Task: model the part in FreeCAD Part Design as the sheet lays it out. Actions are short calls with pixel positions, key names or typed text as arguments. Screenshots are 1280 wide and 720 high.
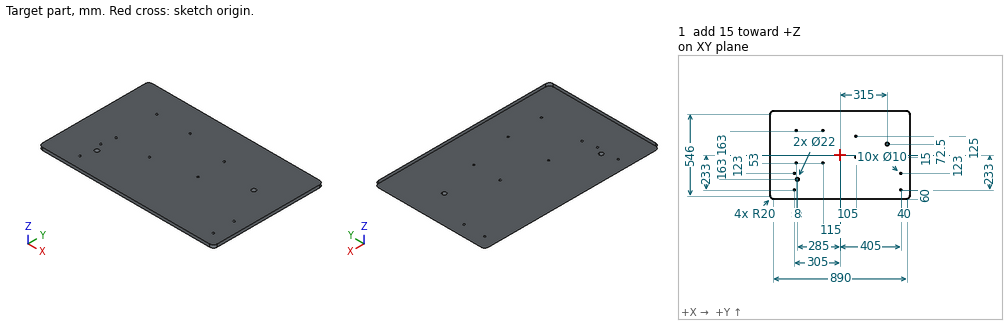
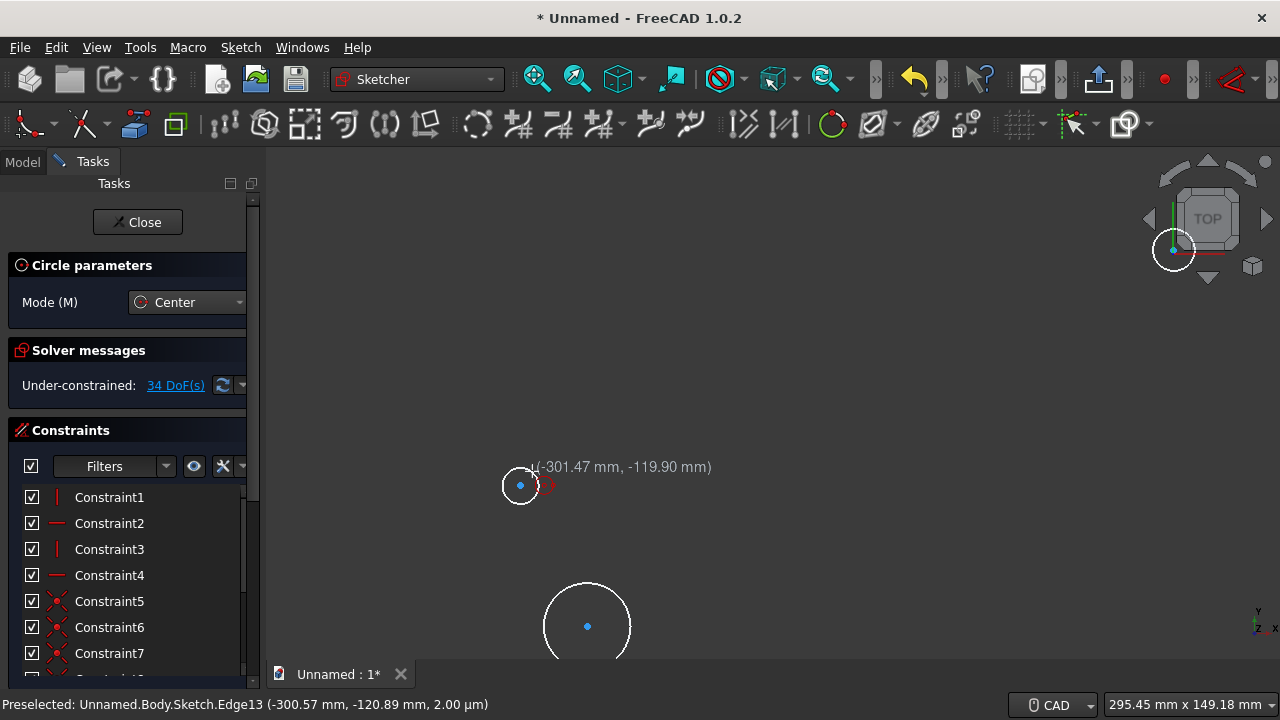
scroll(561, 242, up, 2)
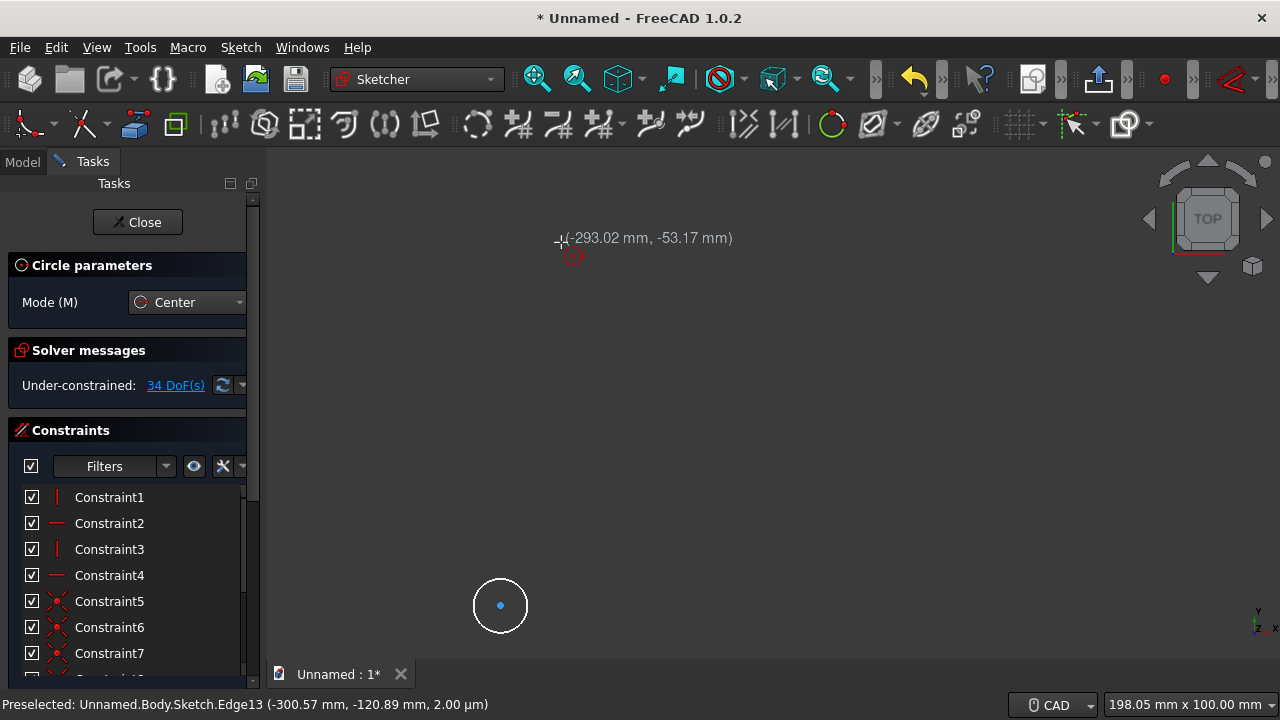
scroll(535, 457, down, 11)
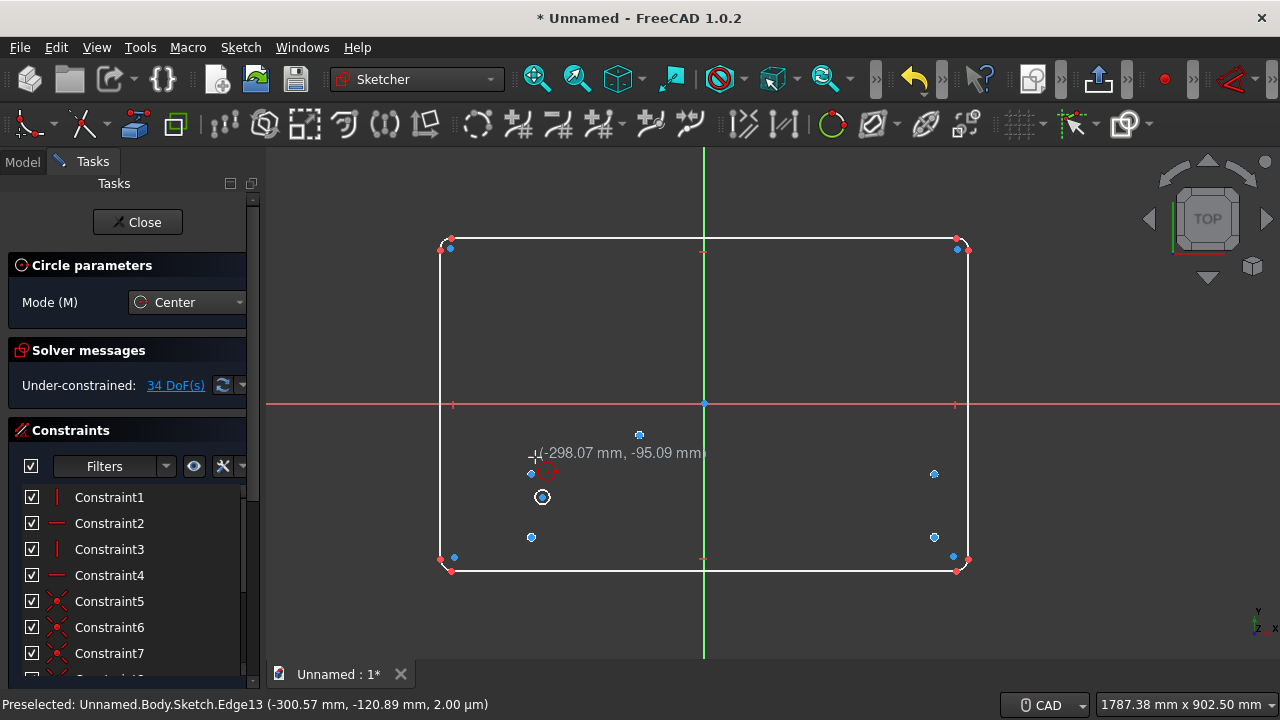
click(538, 434)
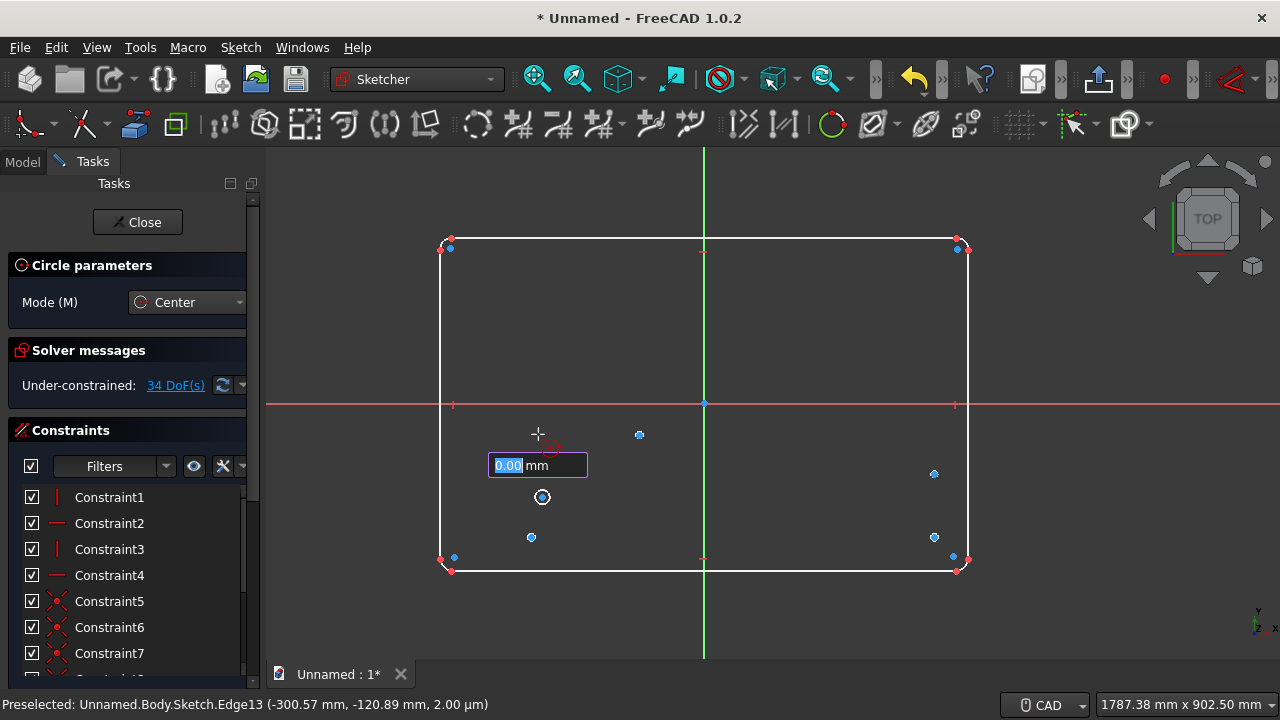
scroll(540, 432, up, 9)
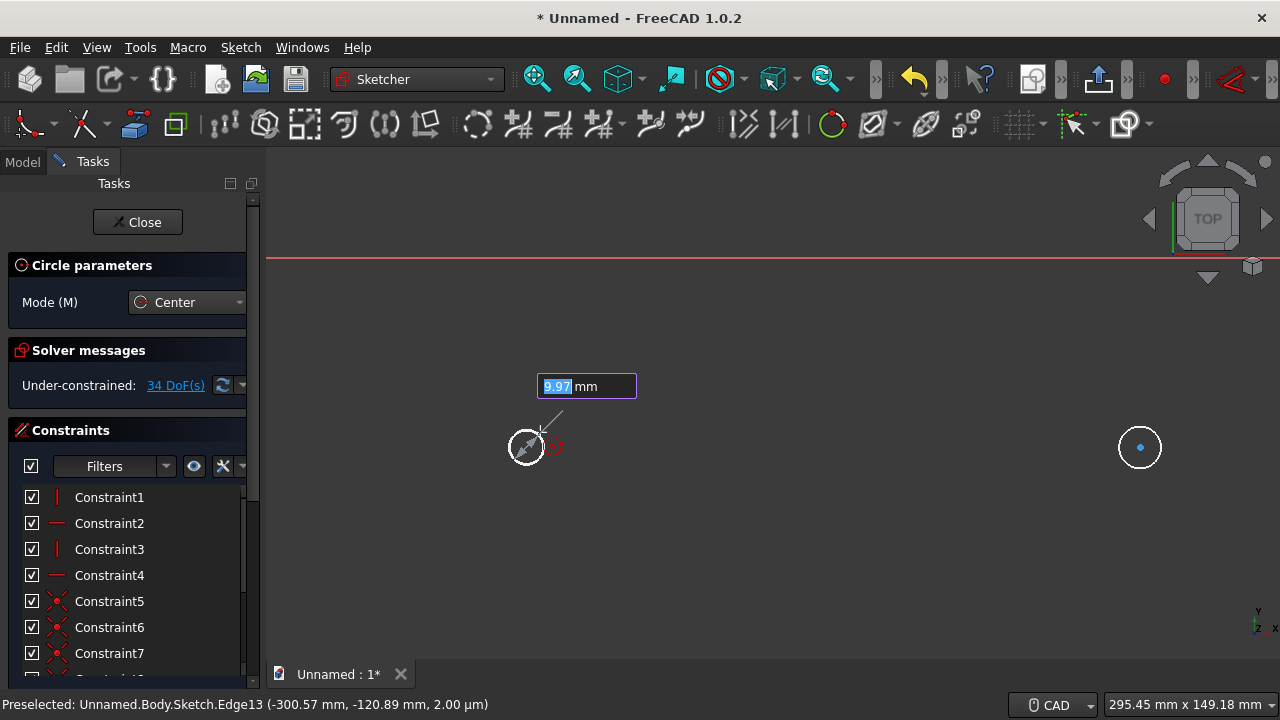
click(539, 428)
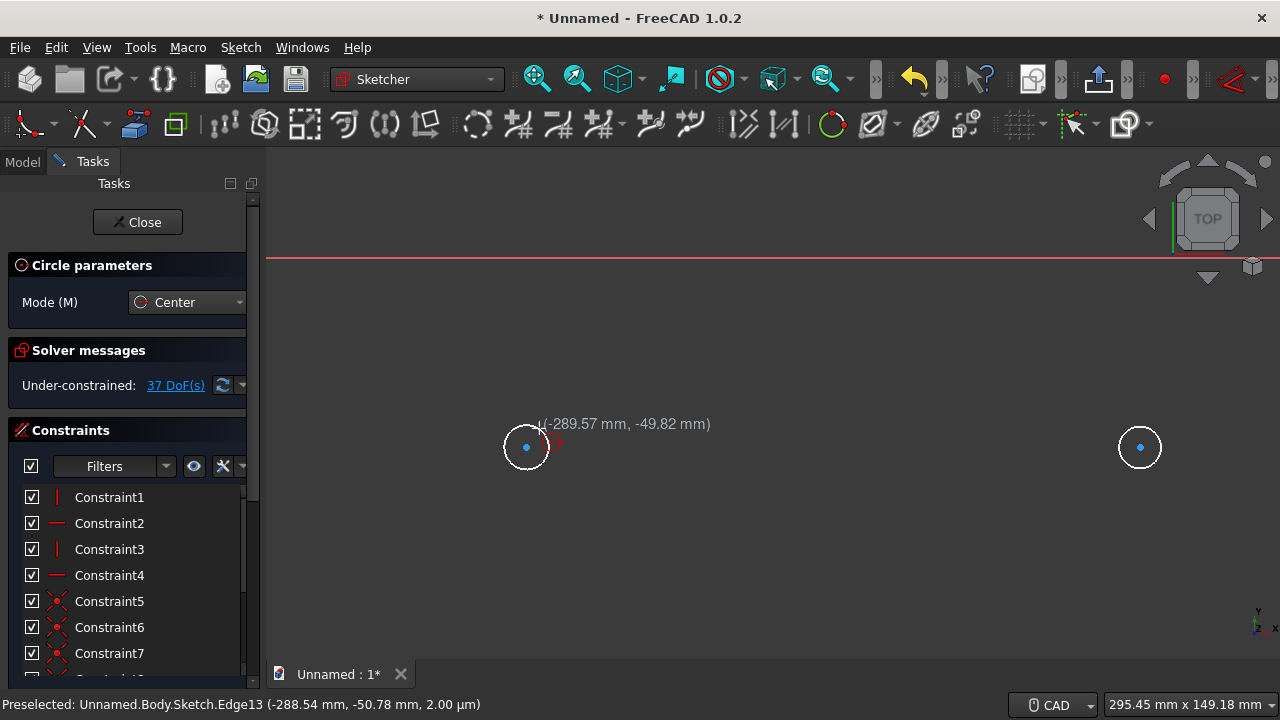
scroll(540, 432, down, 9)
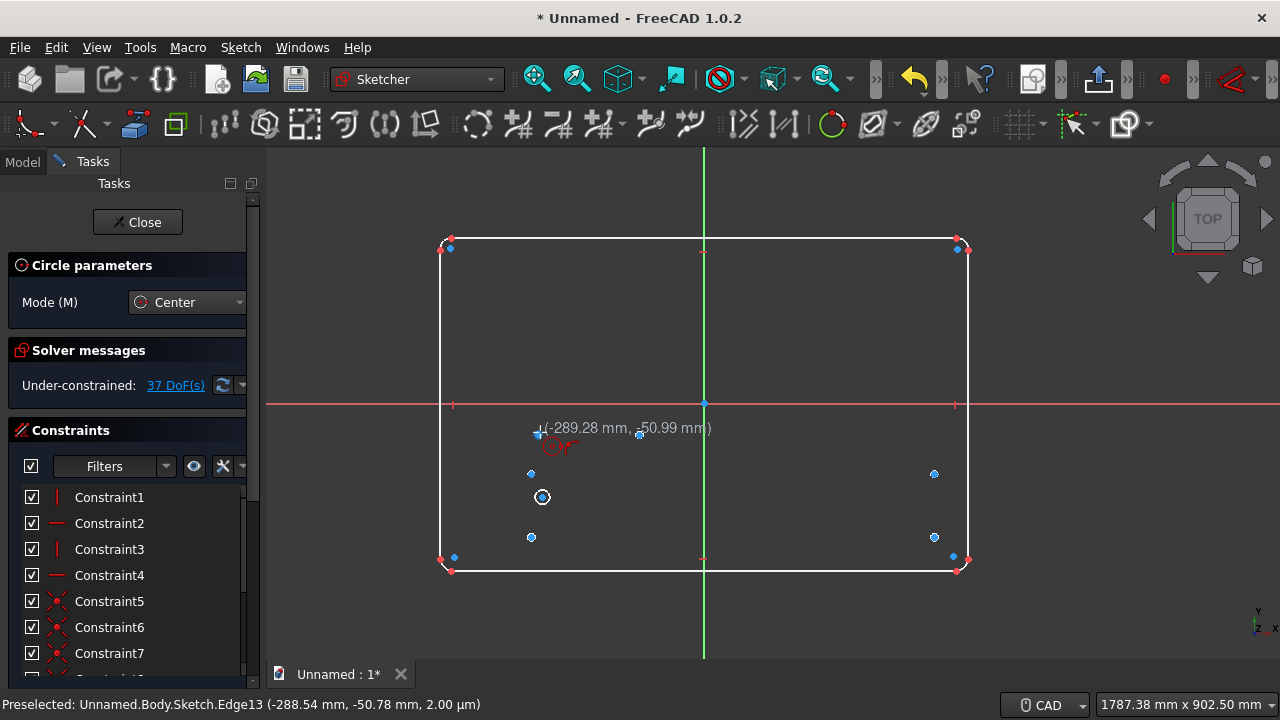
scroll(764, 412, up, 11)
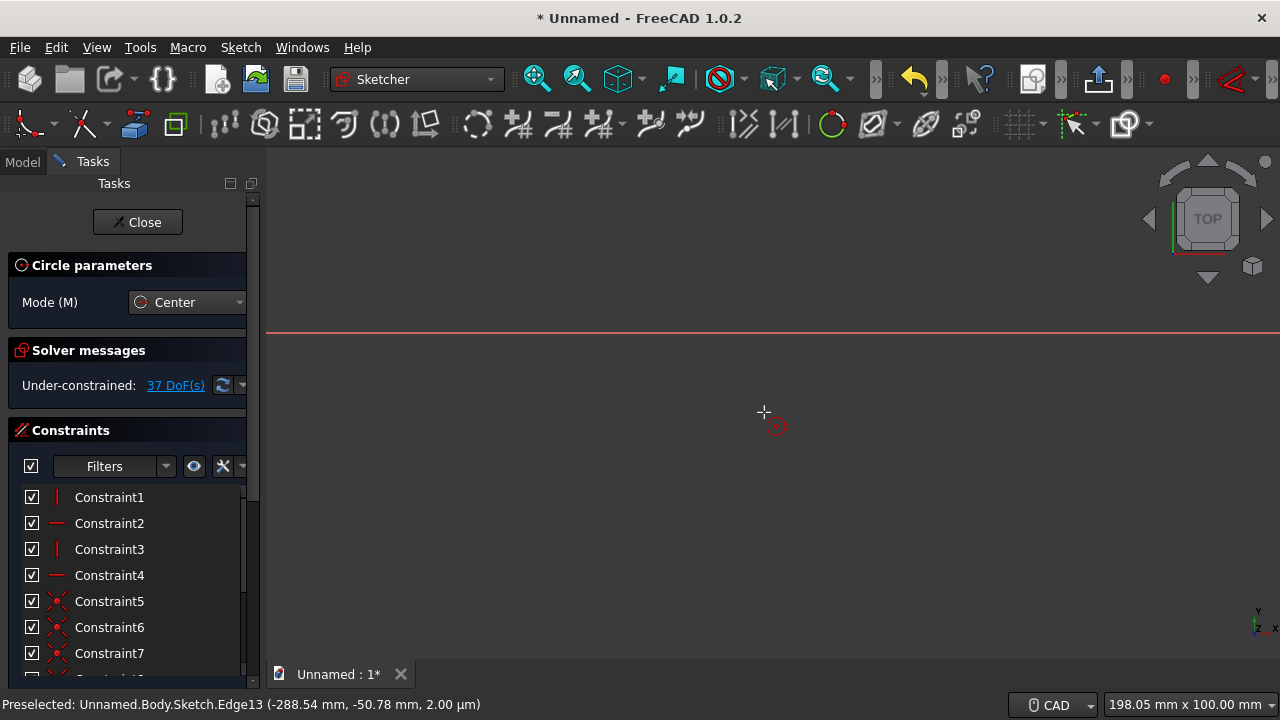
scroll(765, 412, down, 11)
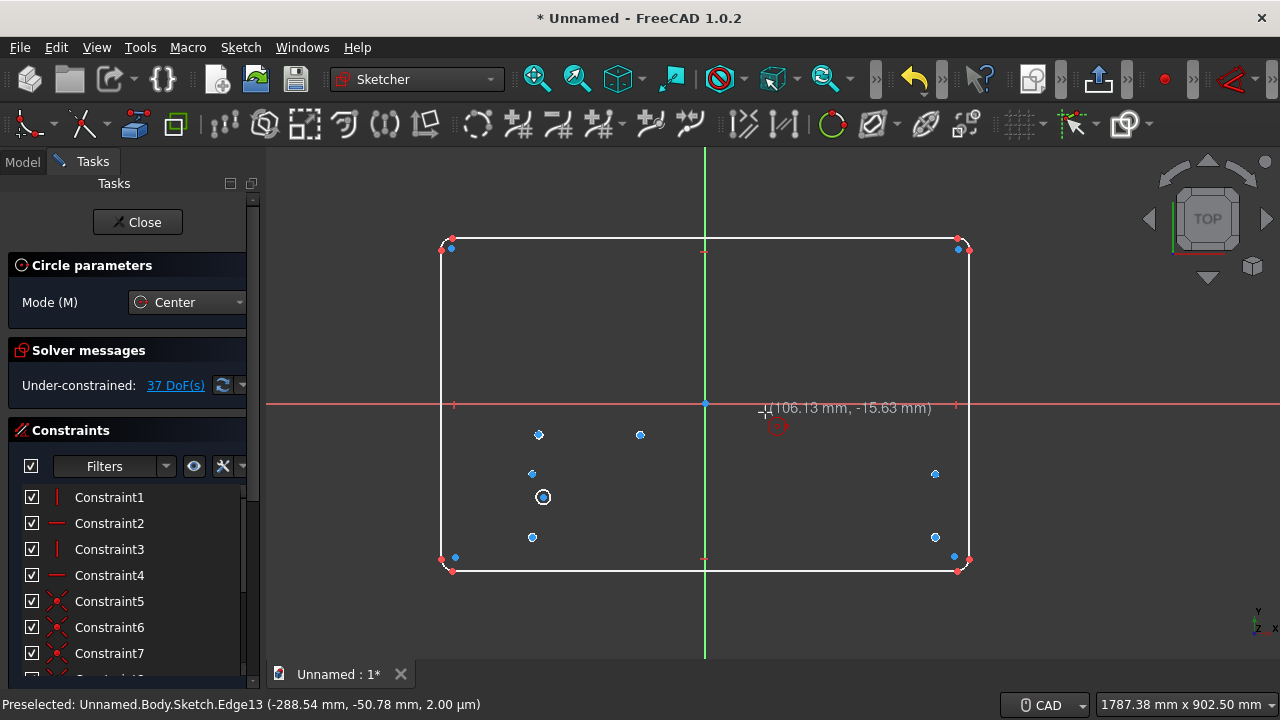
scroll(765, 412, up, 4)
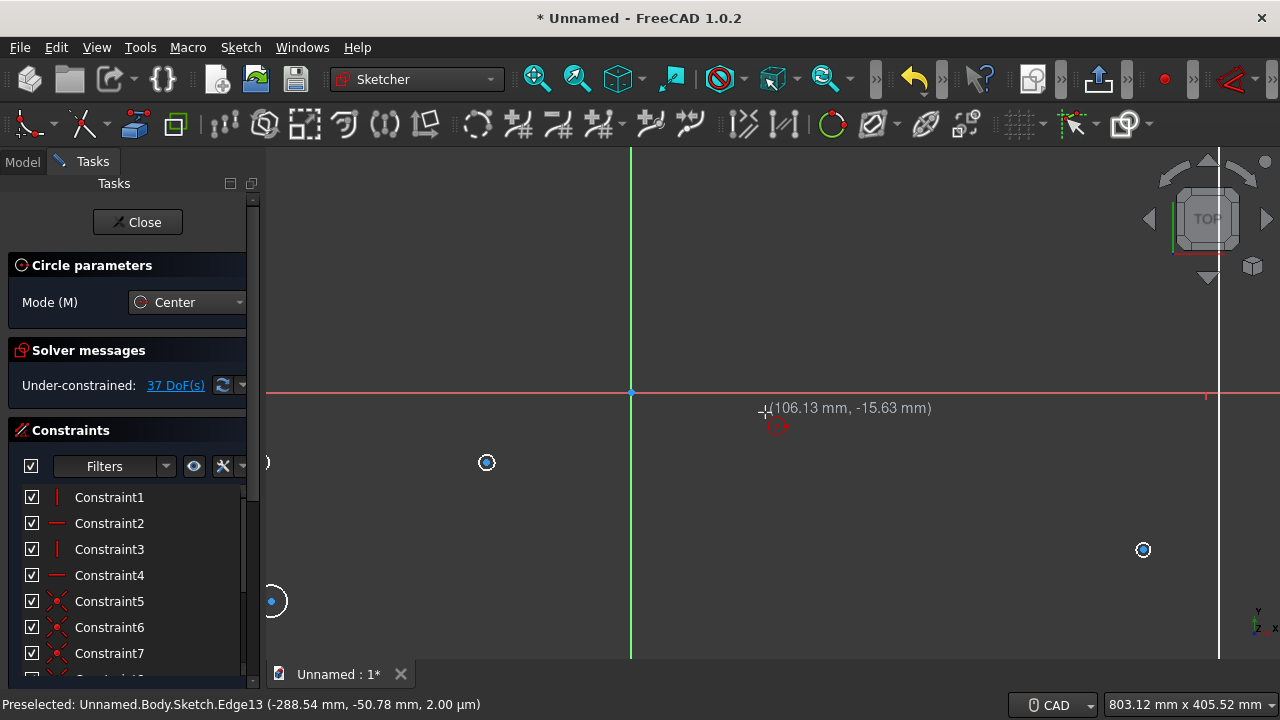
click(764, 412)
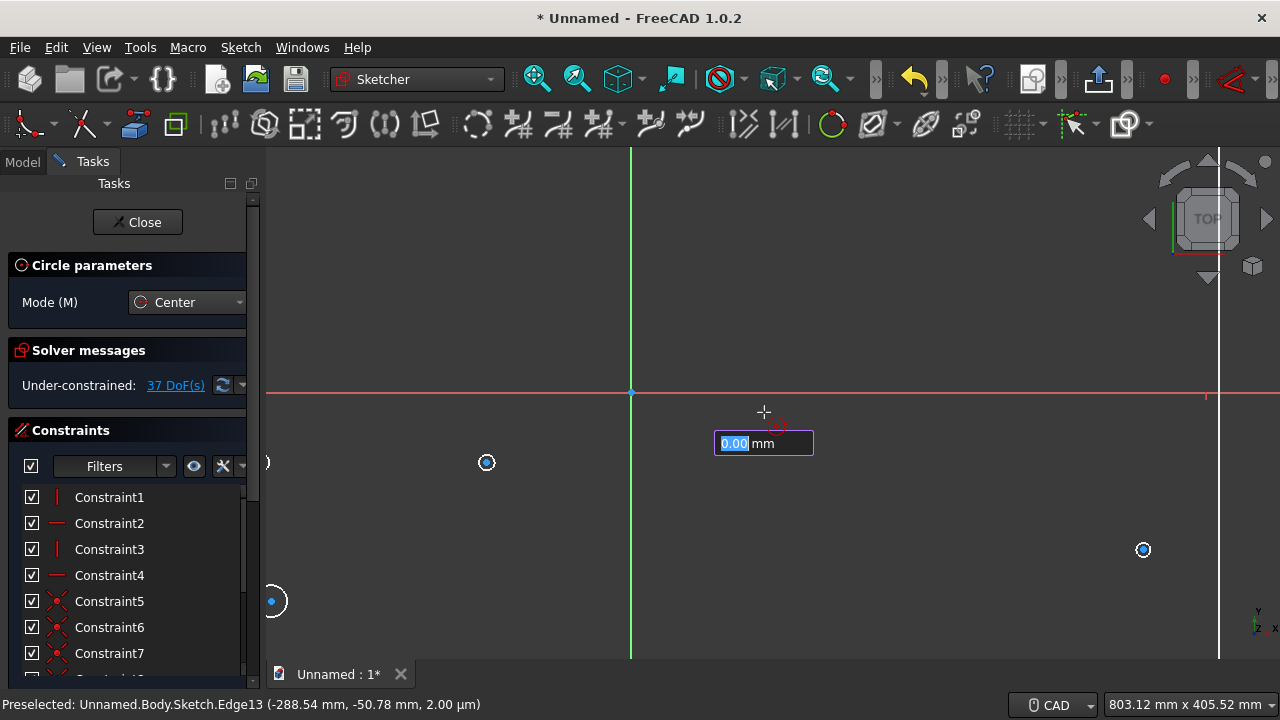
scroll(768, 407, up, 5)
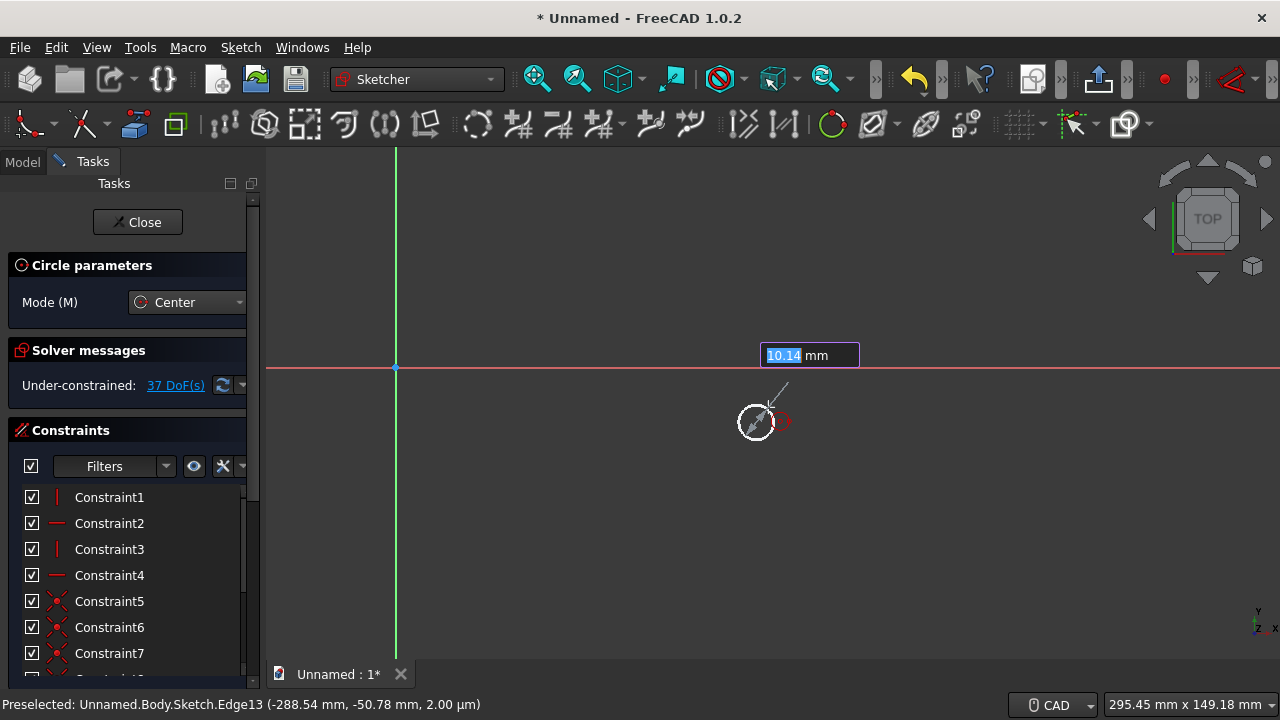
click(768, 407)